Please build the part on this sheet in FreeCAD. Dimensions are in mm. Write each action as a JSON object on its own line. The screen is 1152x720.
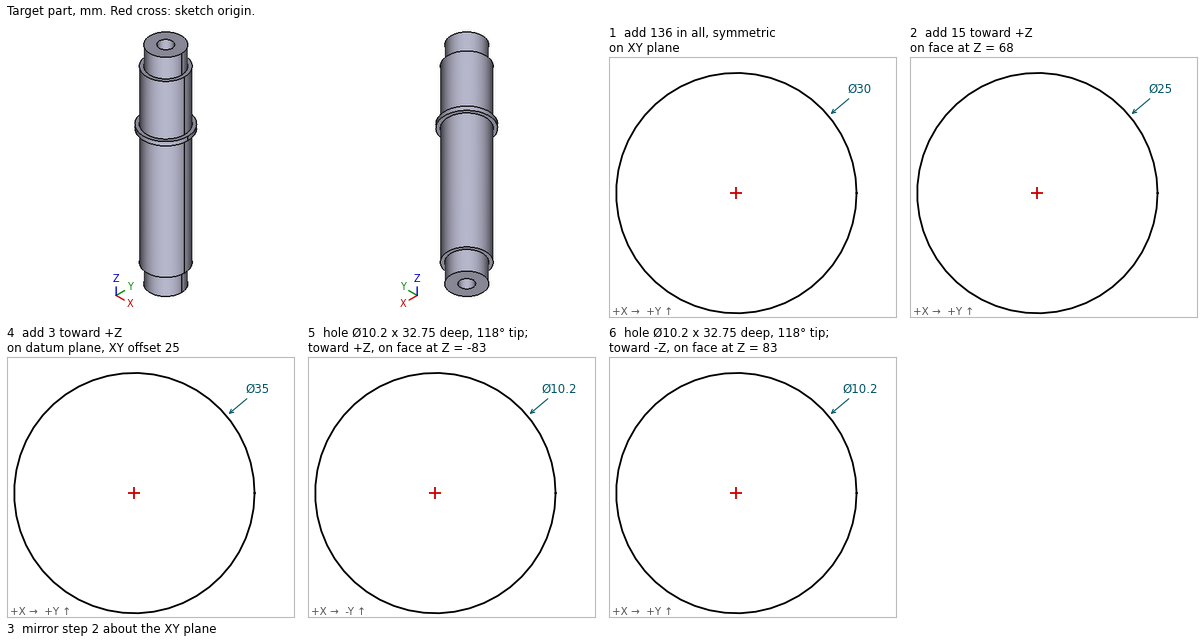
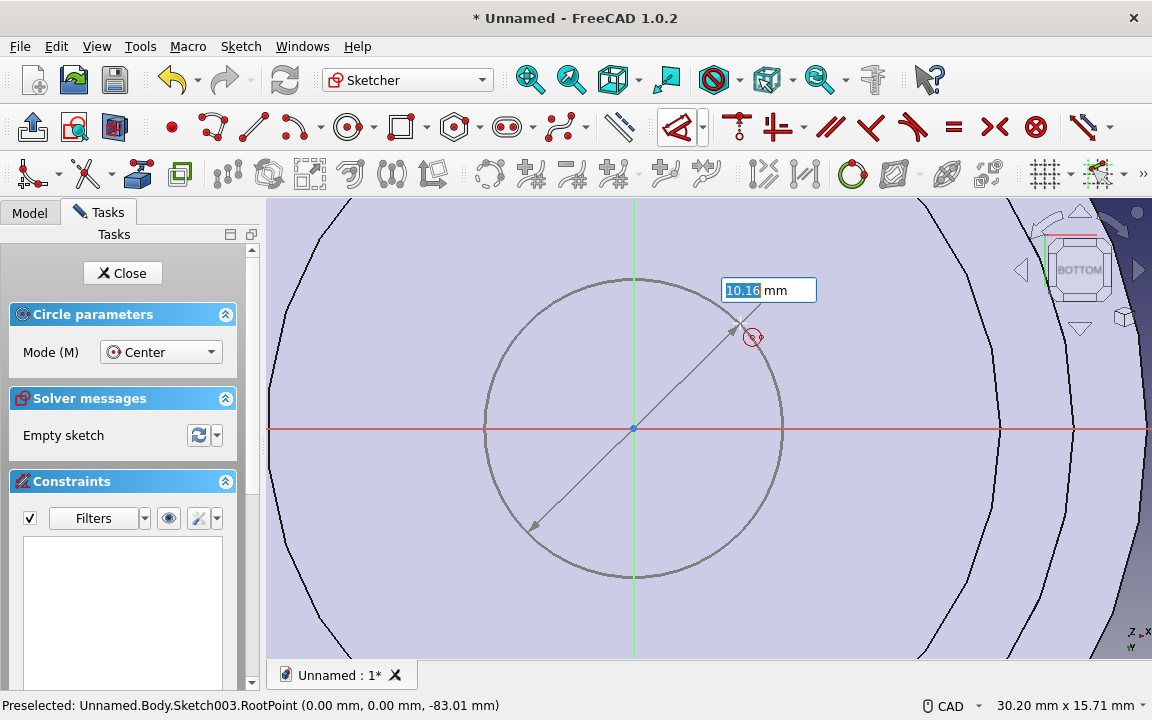
{"action": "type", "text": "10.2"}
{"action": "key", "text": "Return"}
{"action": "key", "text": "Escape"}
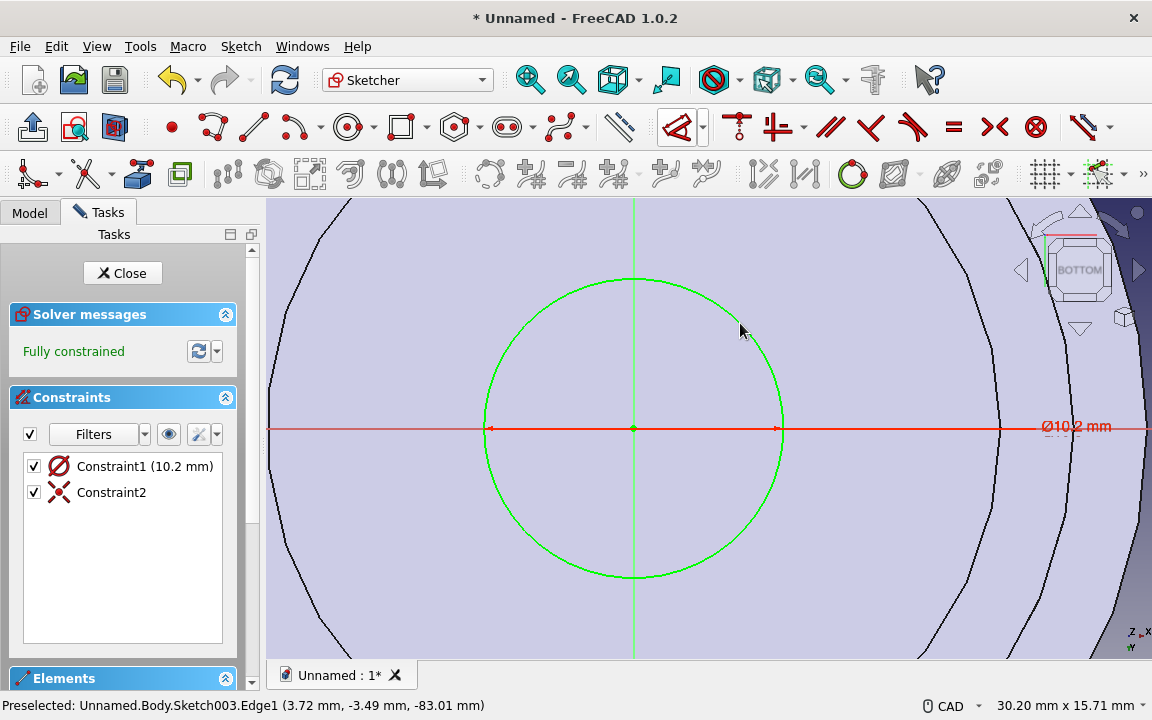
{"action": "left_click", "coordinate": [123, 273]}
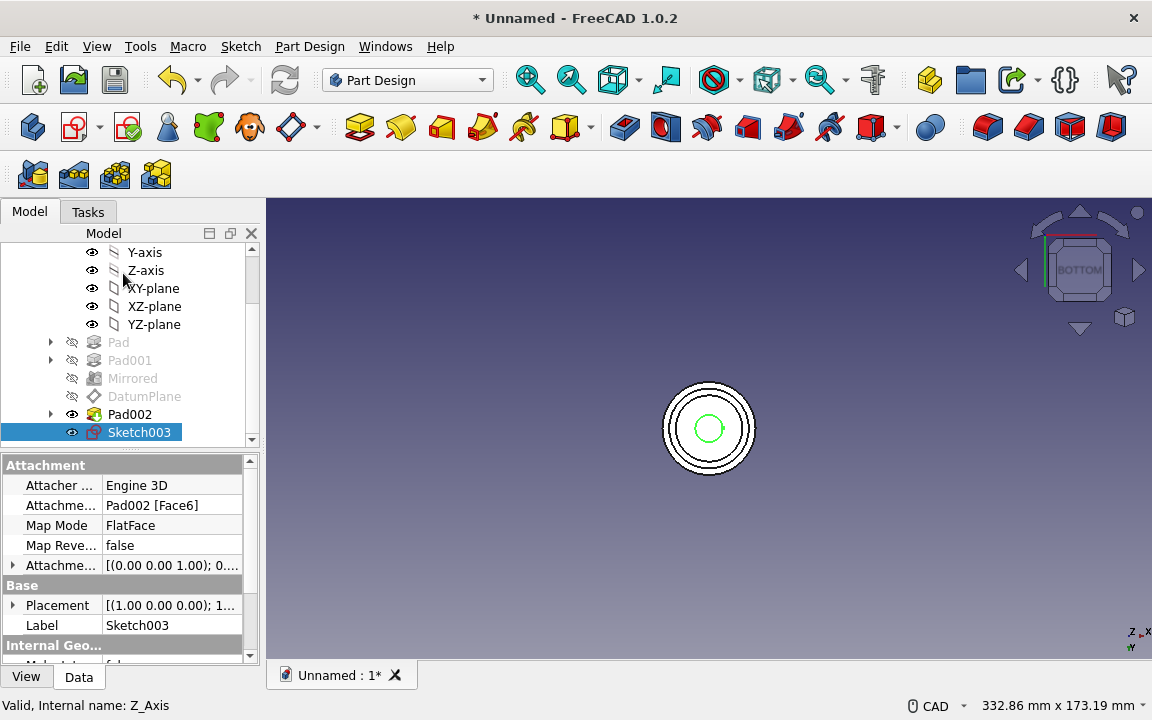
{"action": "left_click", "coordinate": [666, 128]}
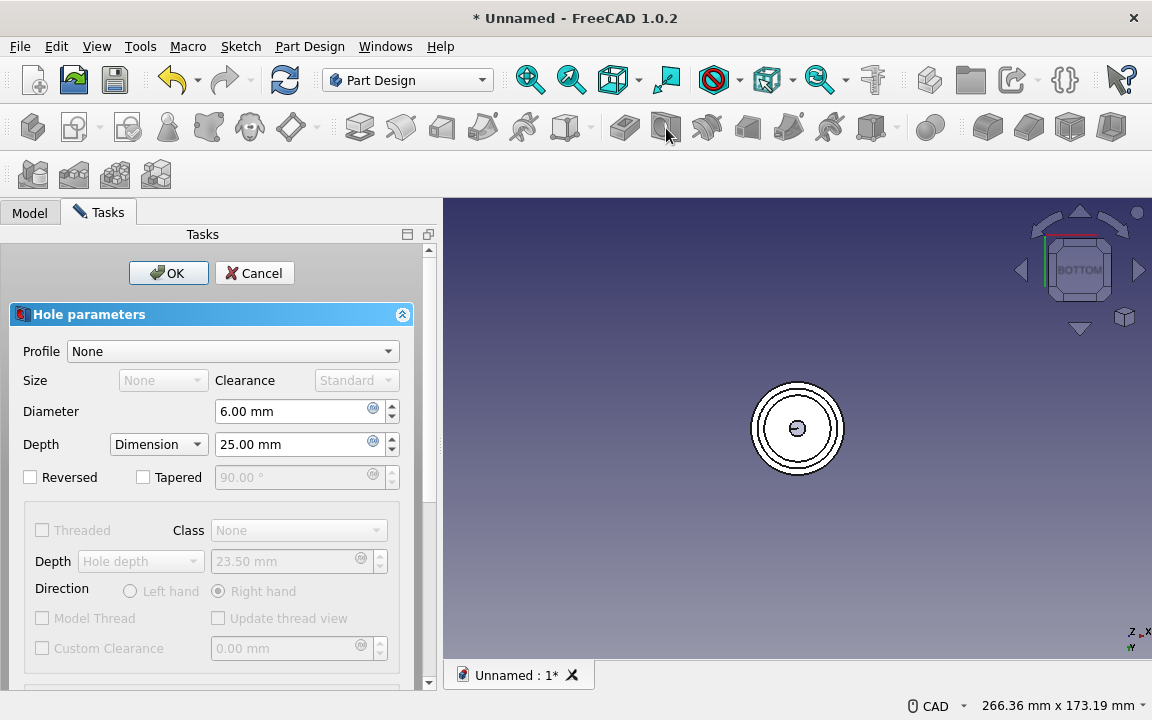
{"action": "triple_click", "coordinate": [300, 412]}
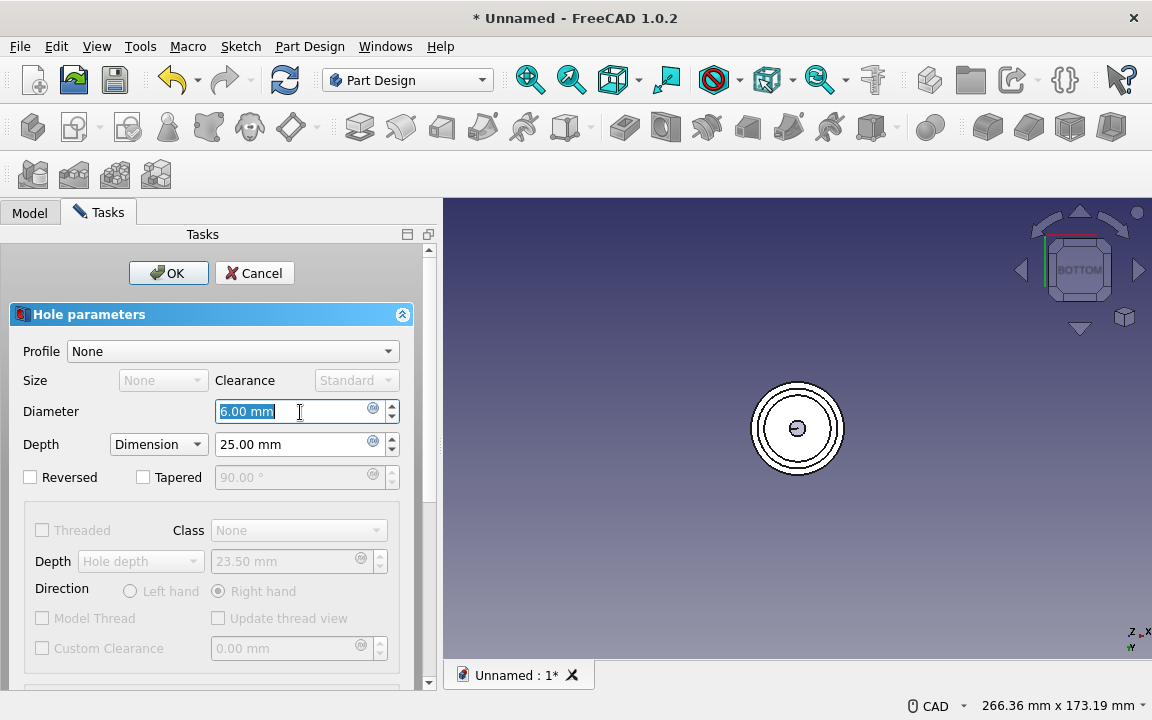
{"action": "type", "text": "10.2"}
{"action": "key", "text": "Tab"}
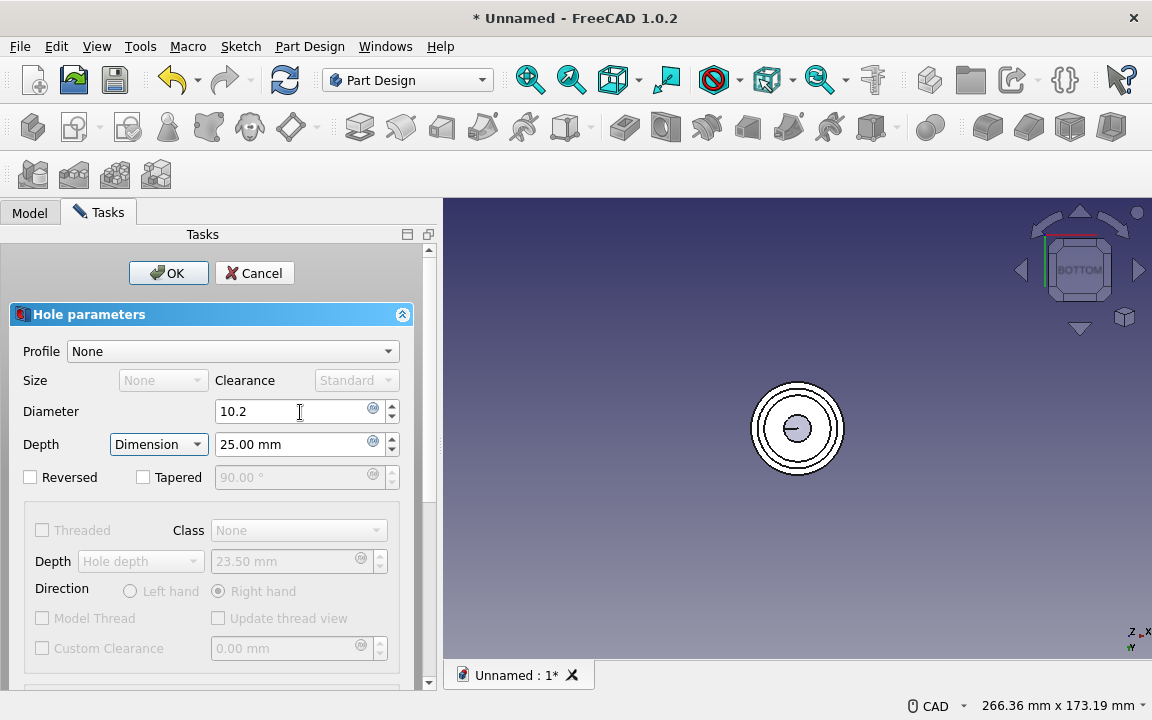
{"action": "triple_click", "coordinate": [300, 444]}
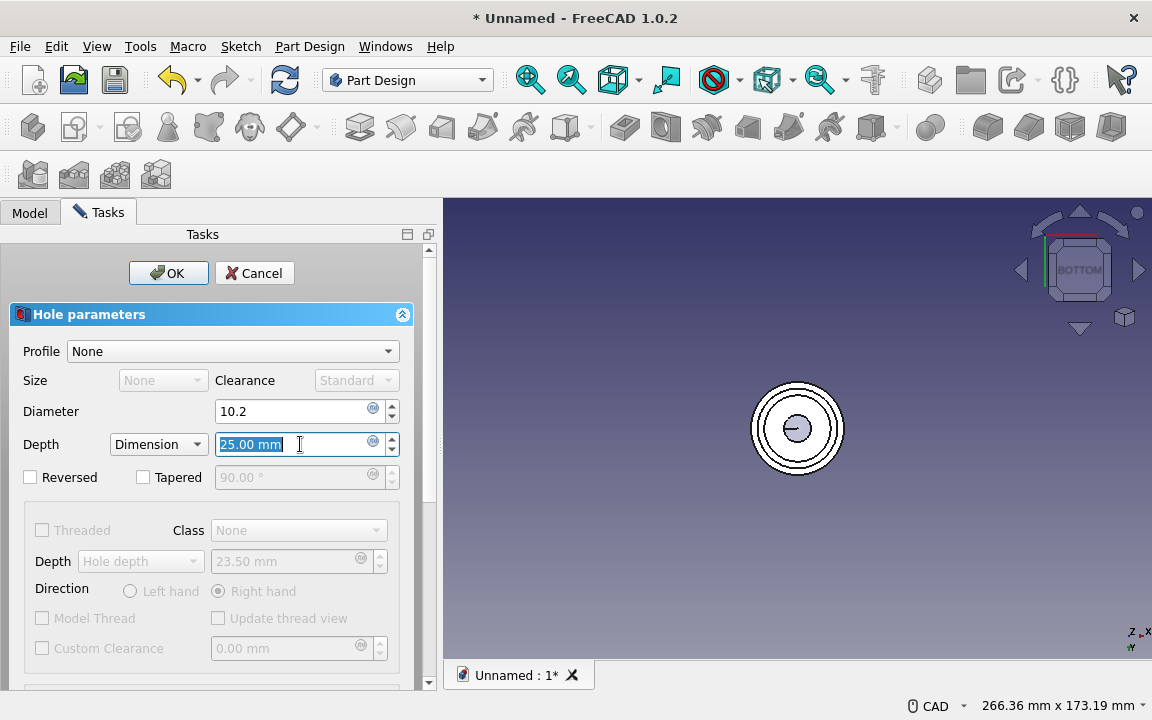
{"action": "type", "text": "32.75"}
{"action": "key", "text": "Tab"}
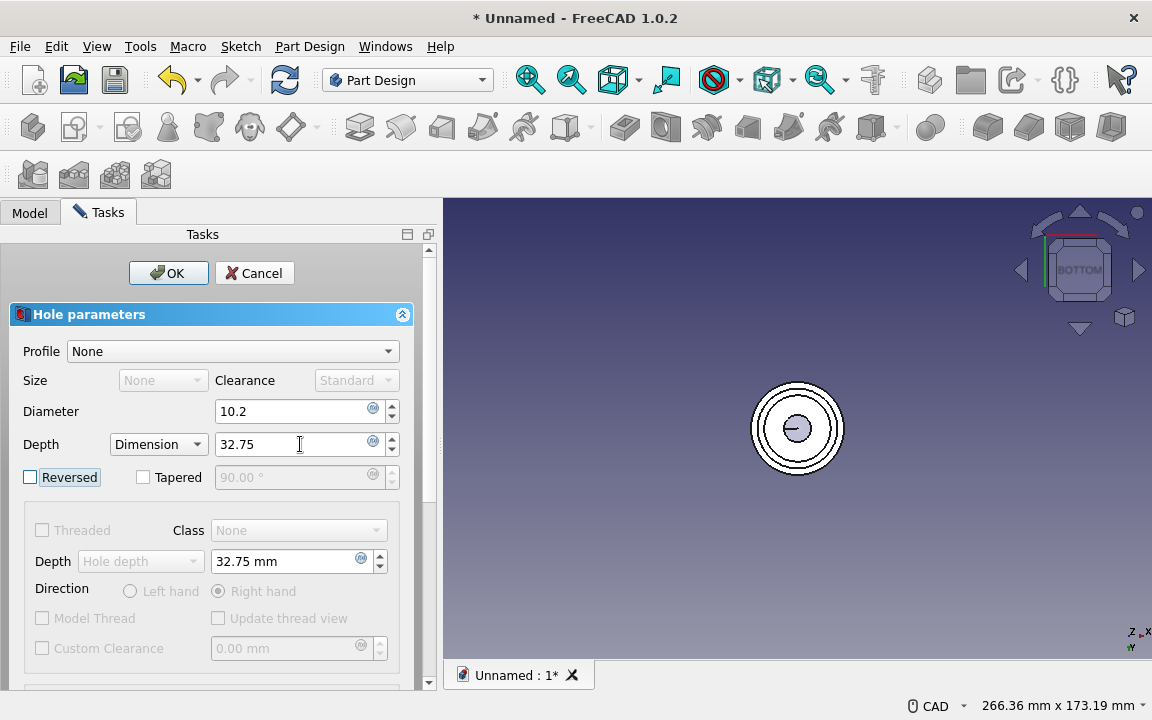
{"action": "left_click", "coordinate": [169, 273]}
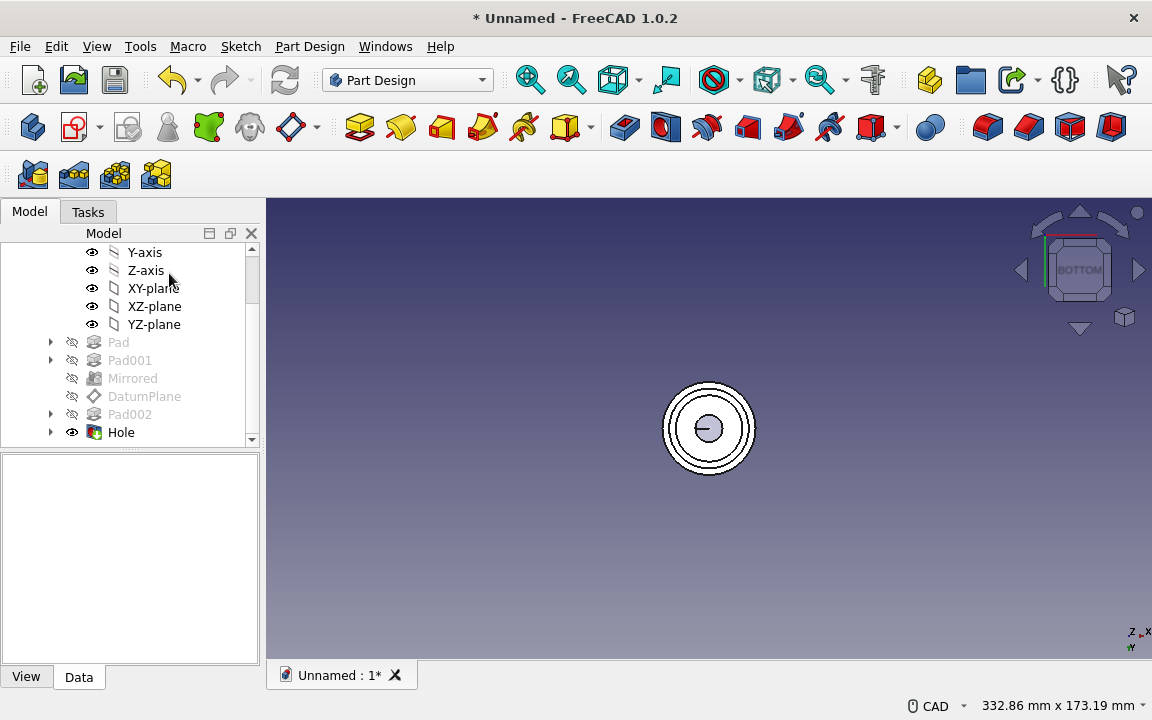
{"action": "left_click", "coordinate": [531, 80]}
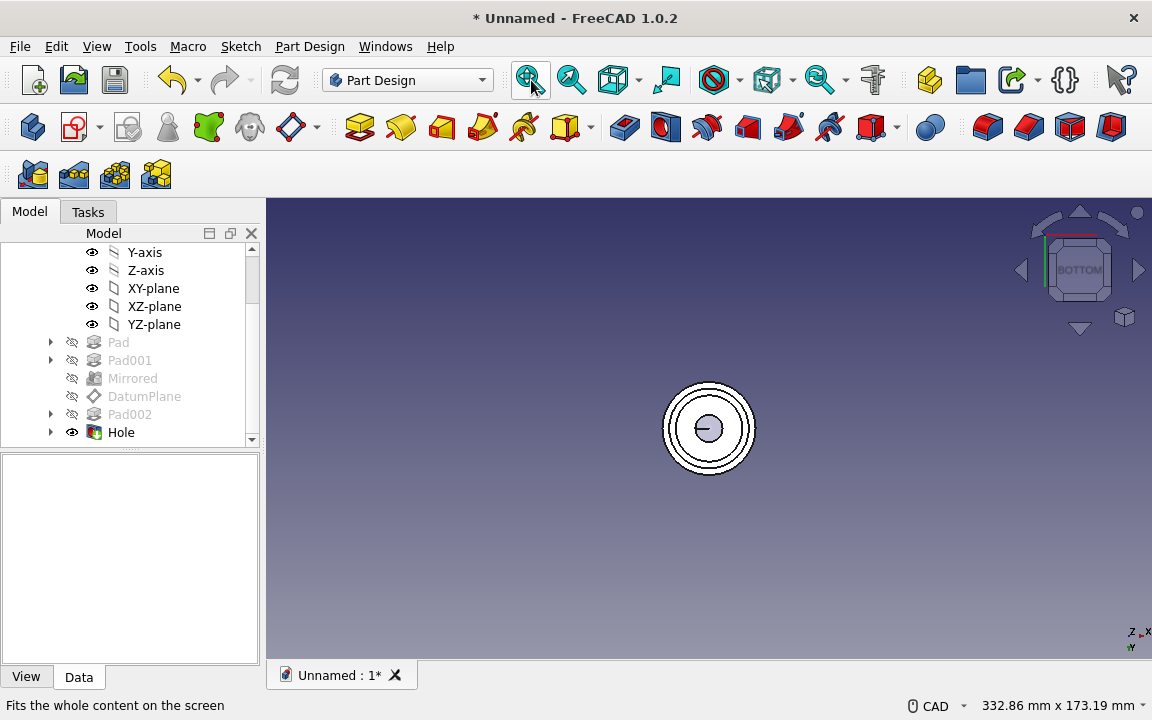
{"action": "key", "text": "0"}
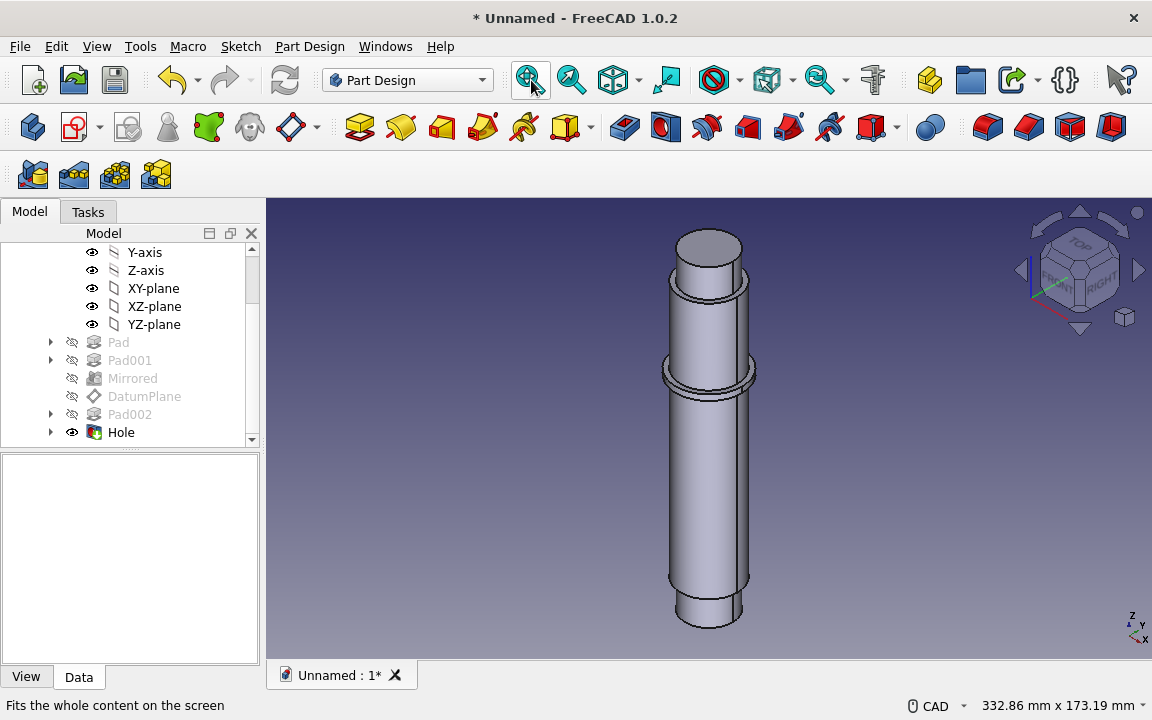
{"action": "left_click", "coordinate": [709, 247]}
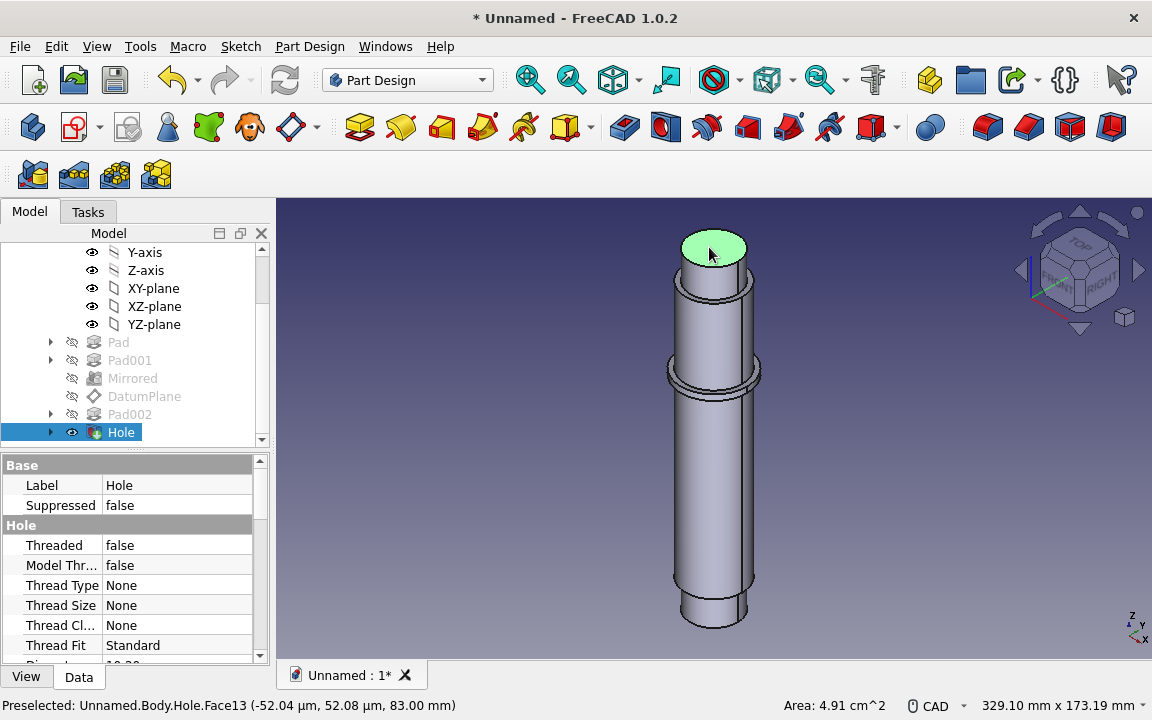
{"action": "left_click", "coordinate": [74, 128]}